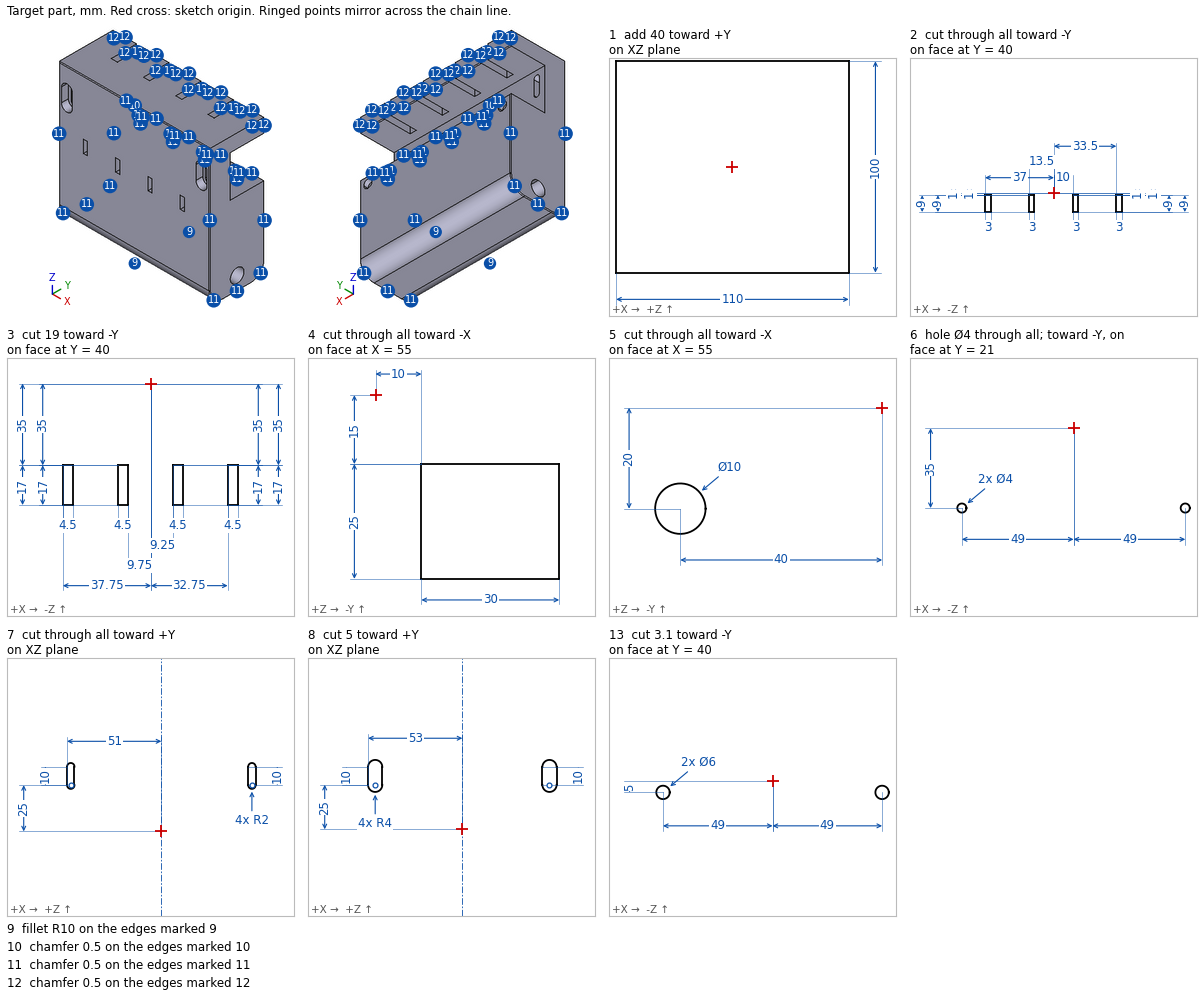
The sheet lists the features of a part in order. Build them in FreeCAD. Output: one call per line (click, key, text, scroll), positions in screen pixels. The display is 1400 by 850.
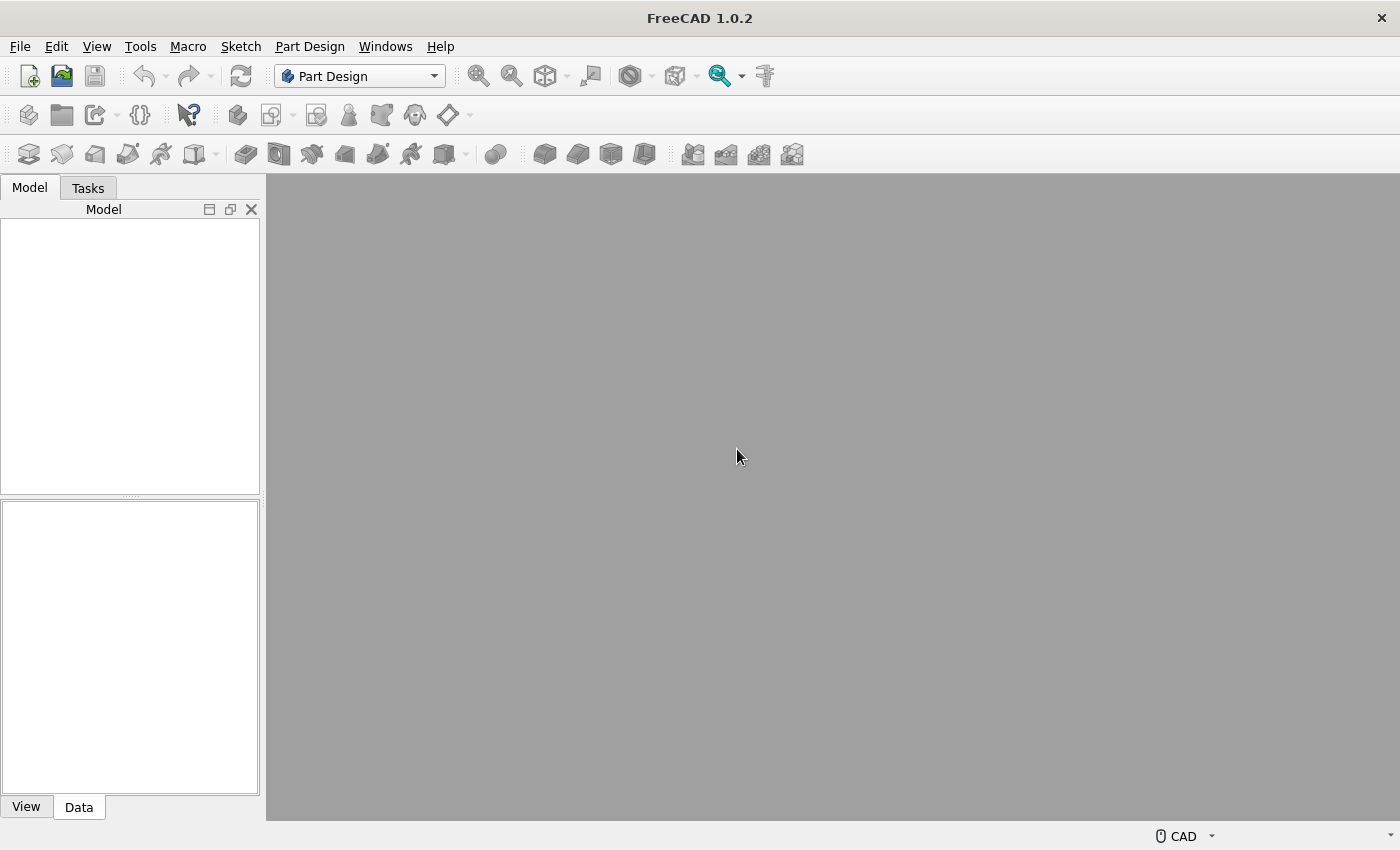
key(ctrl+n)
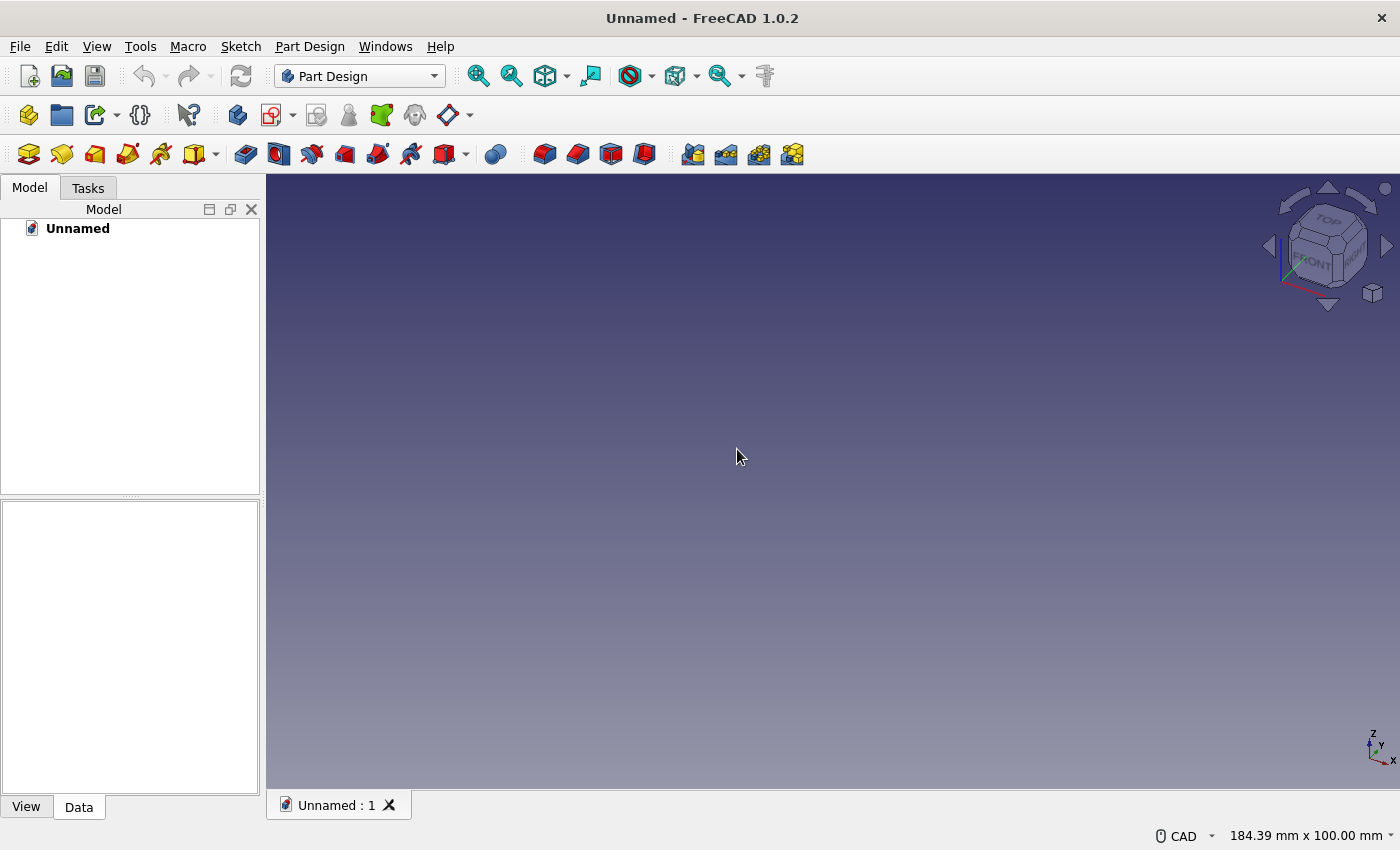
click(270, 116)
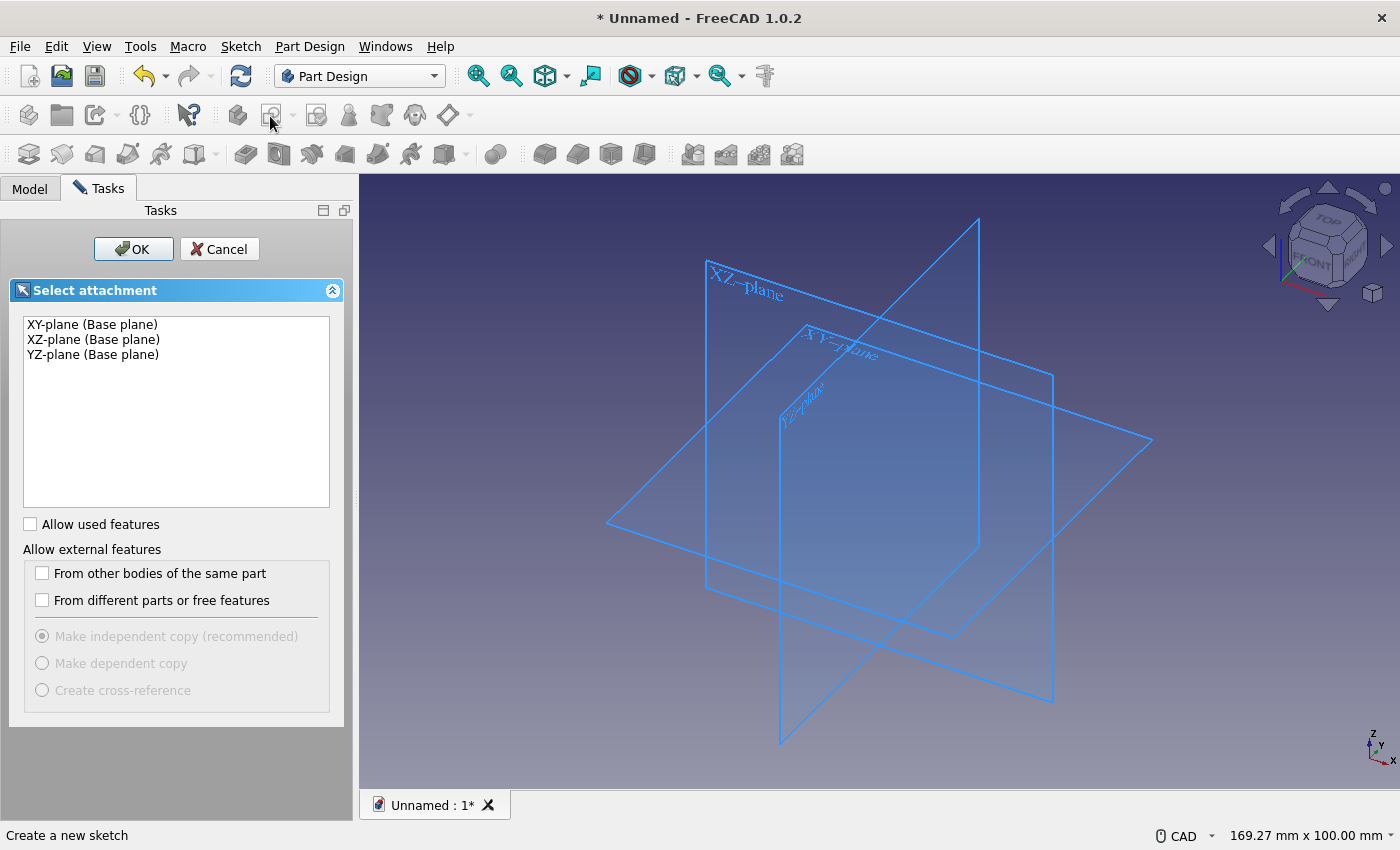
click(84, 340)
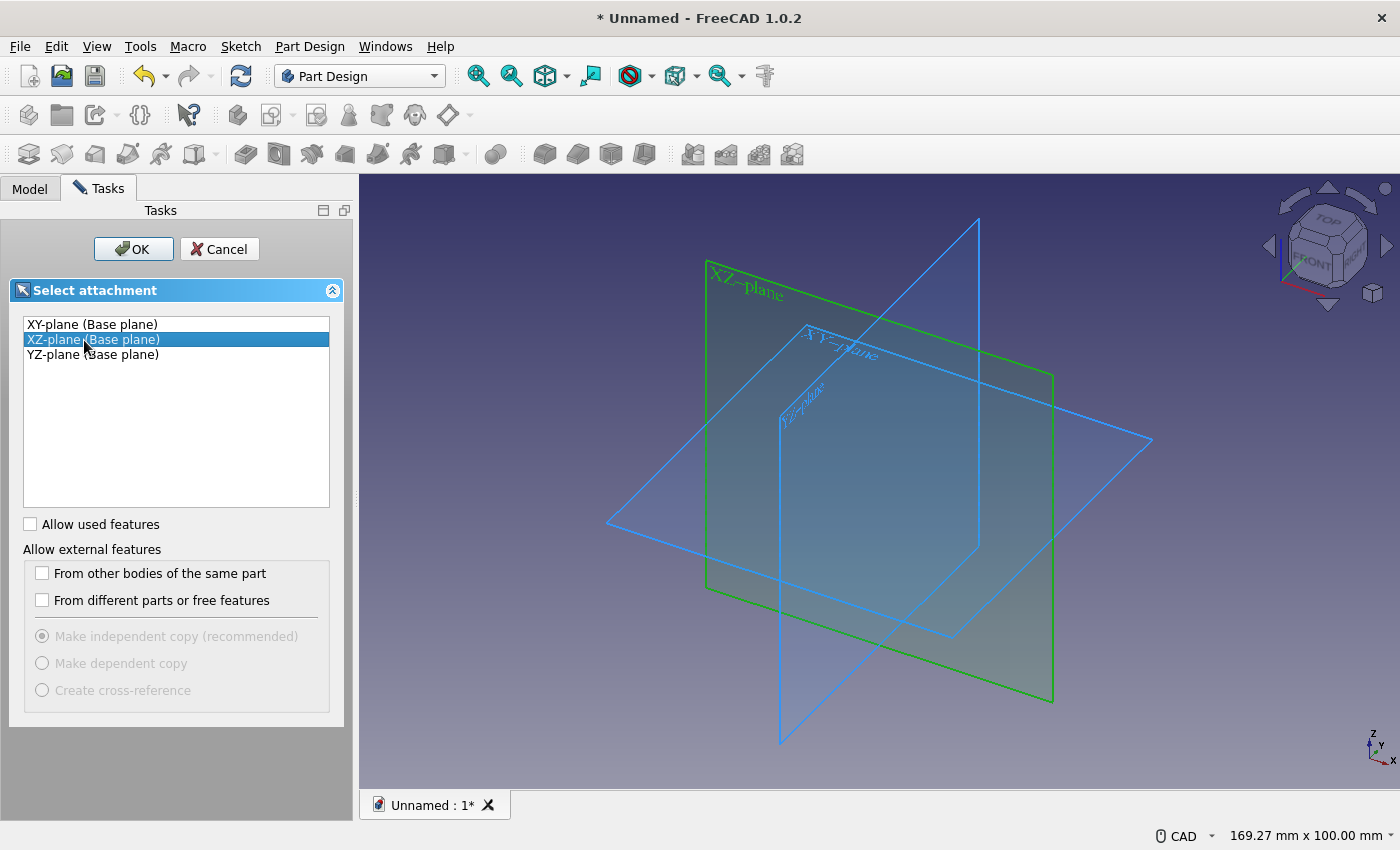
click(134, 249)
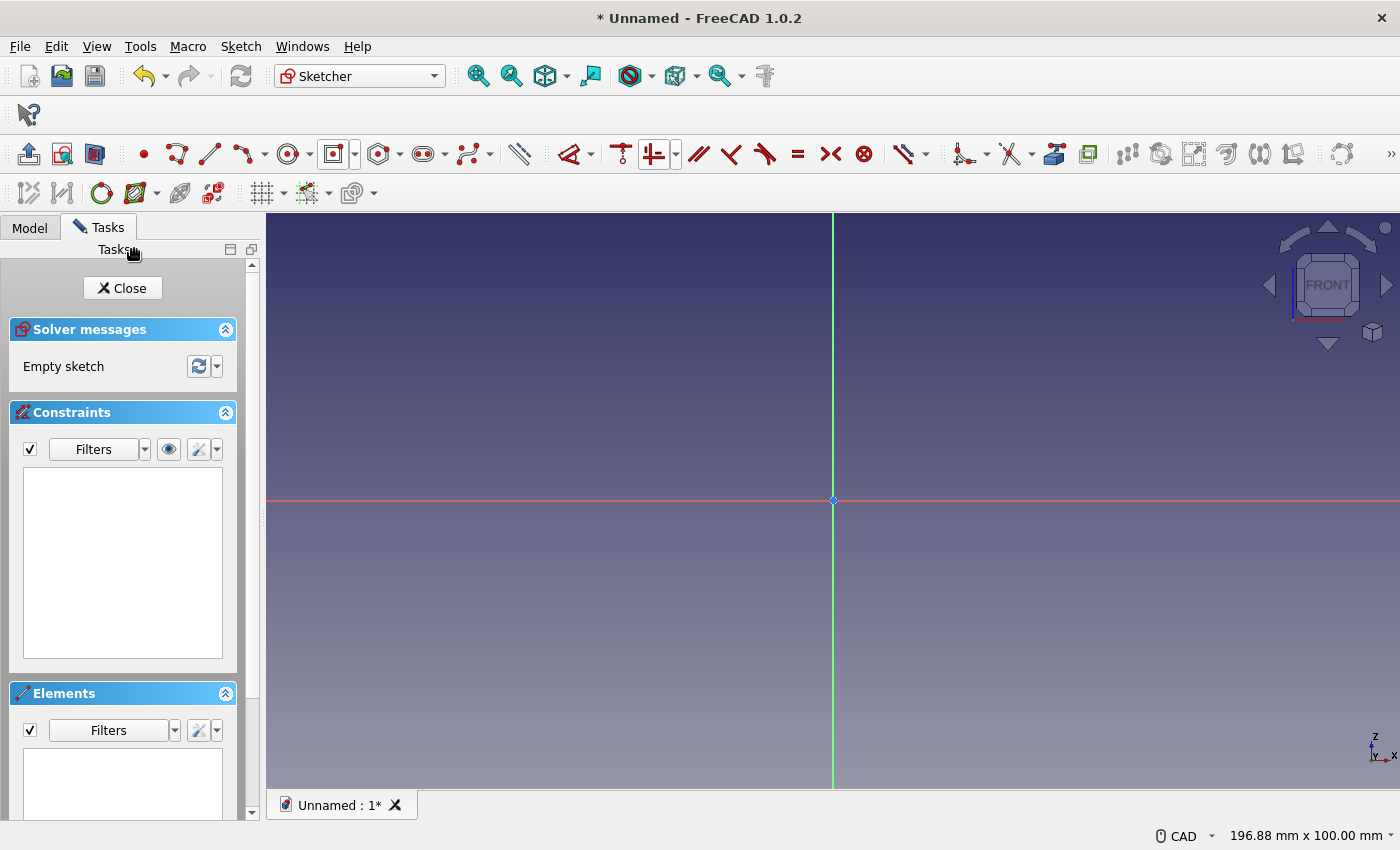
scroll(625, 501, down, 2)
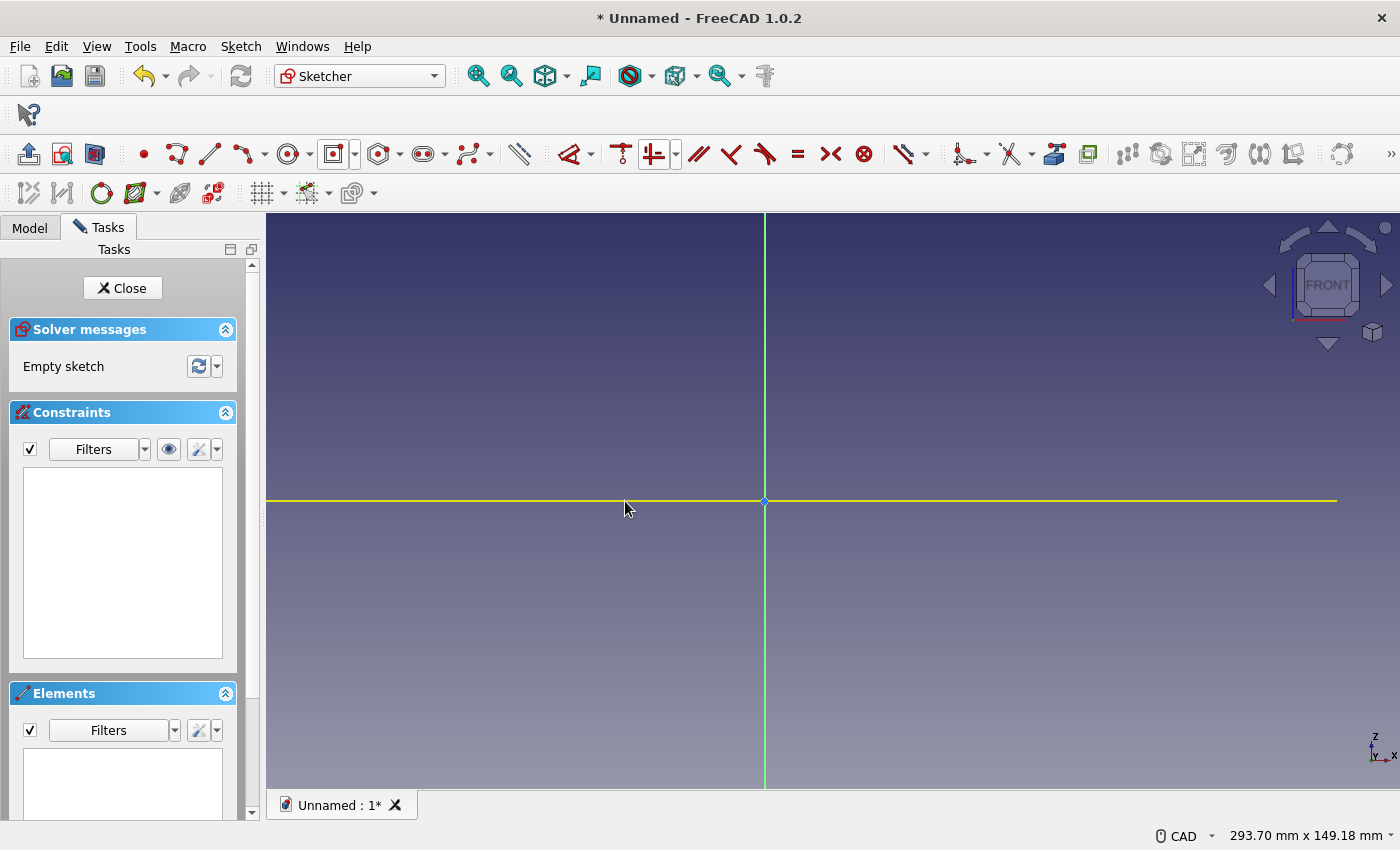
key(g)
key(v)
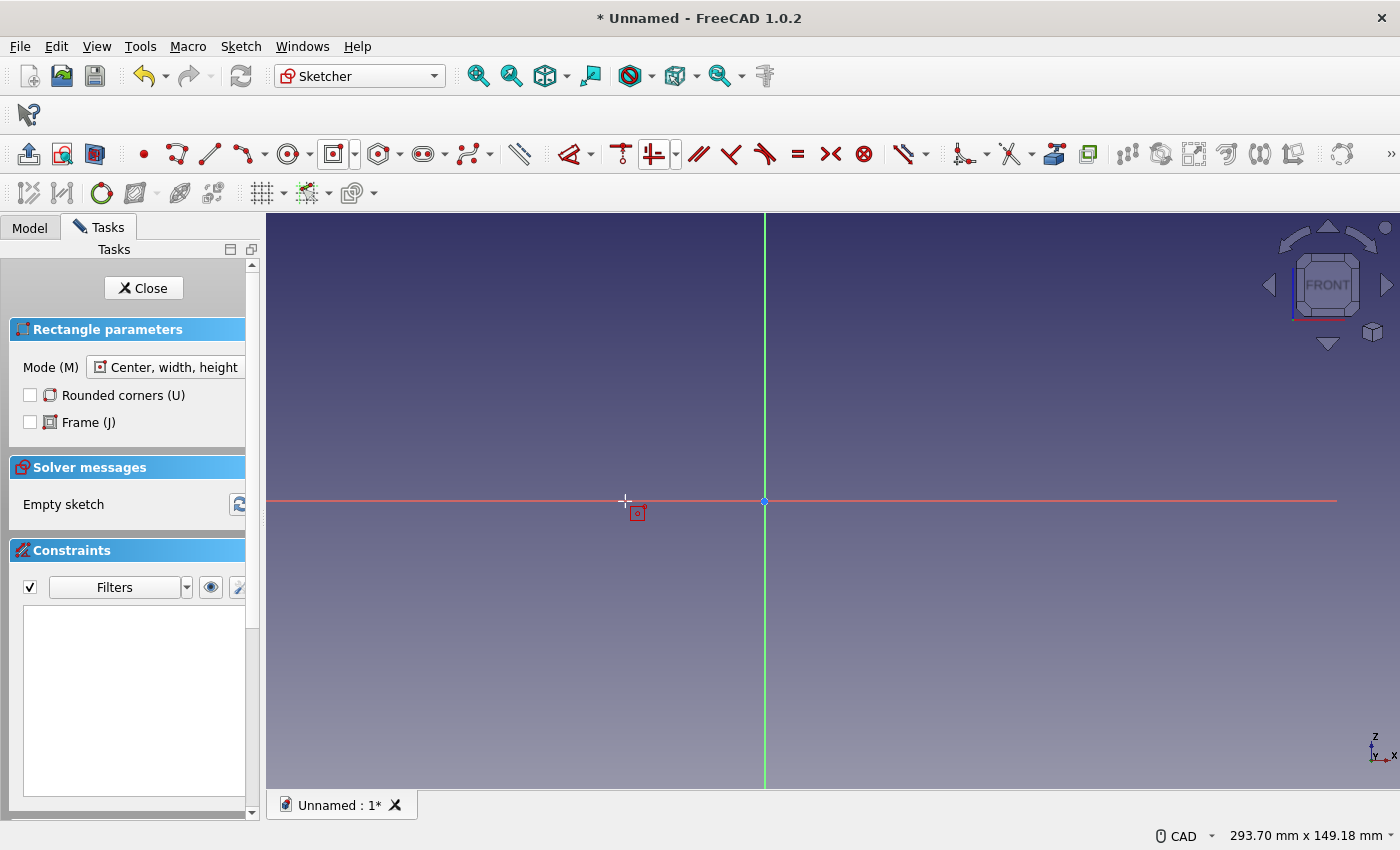
click(765, 501)
click(977, 308)
key(Escape)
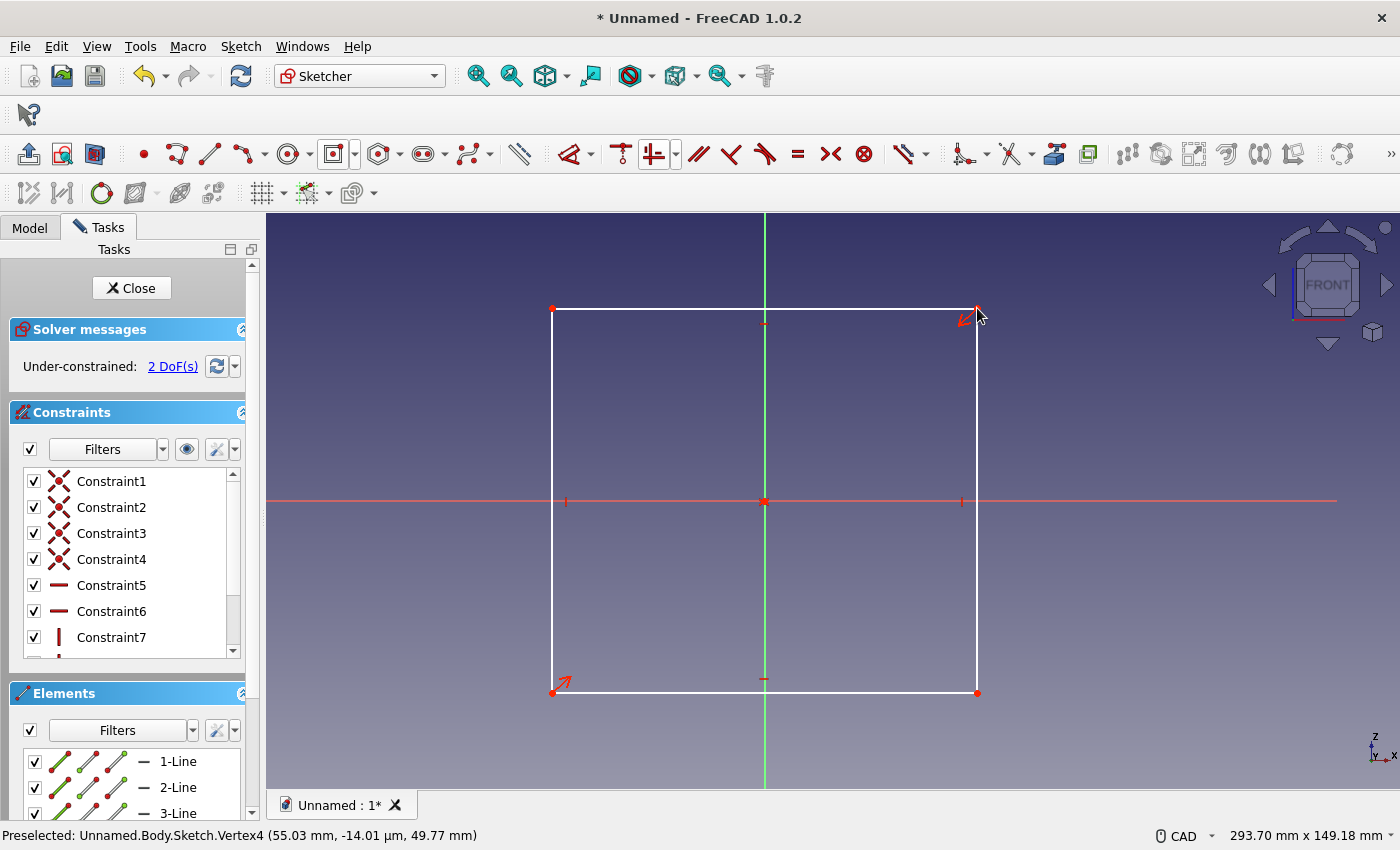
key(d)